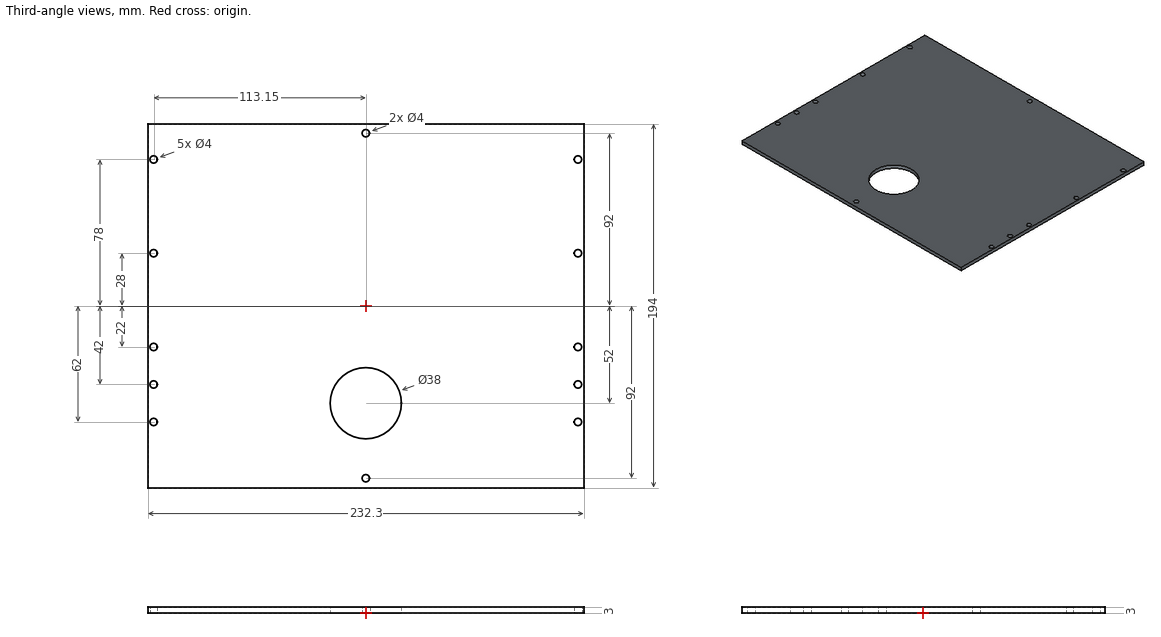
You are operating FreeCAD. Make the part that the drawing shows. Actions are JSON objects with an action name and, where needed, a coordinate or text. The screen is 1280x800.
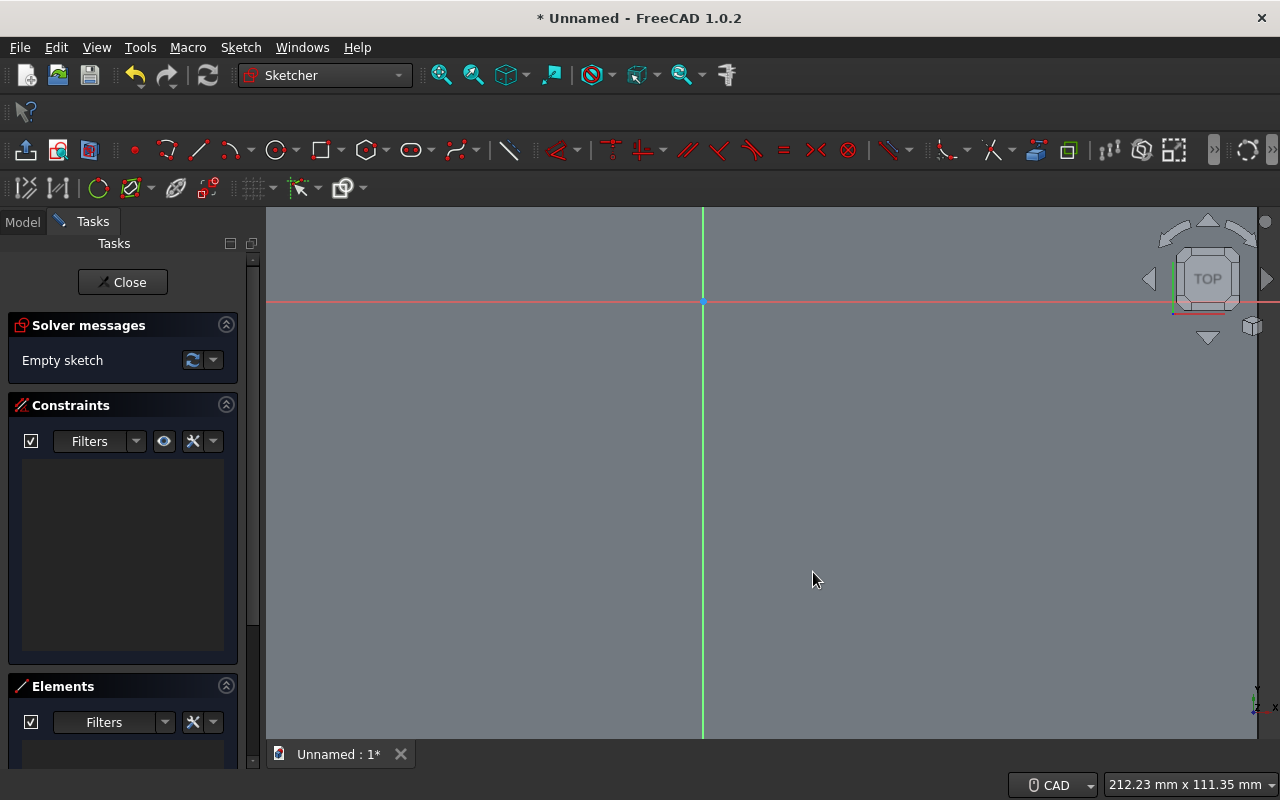
{"action": "left_click", "coordinate": [276, 150]}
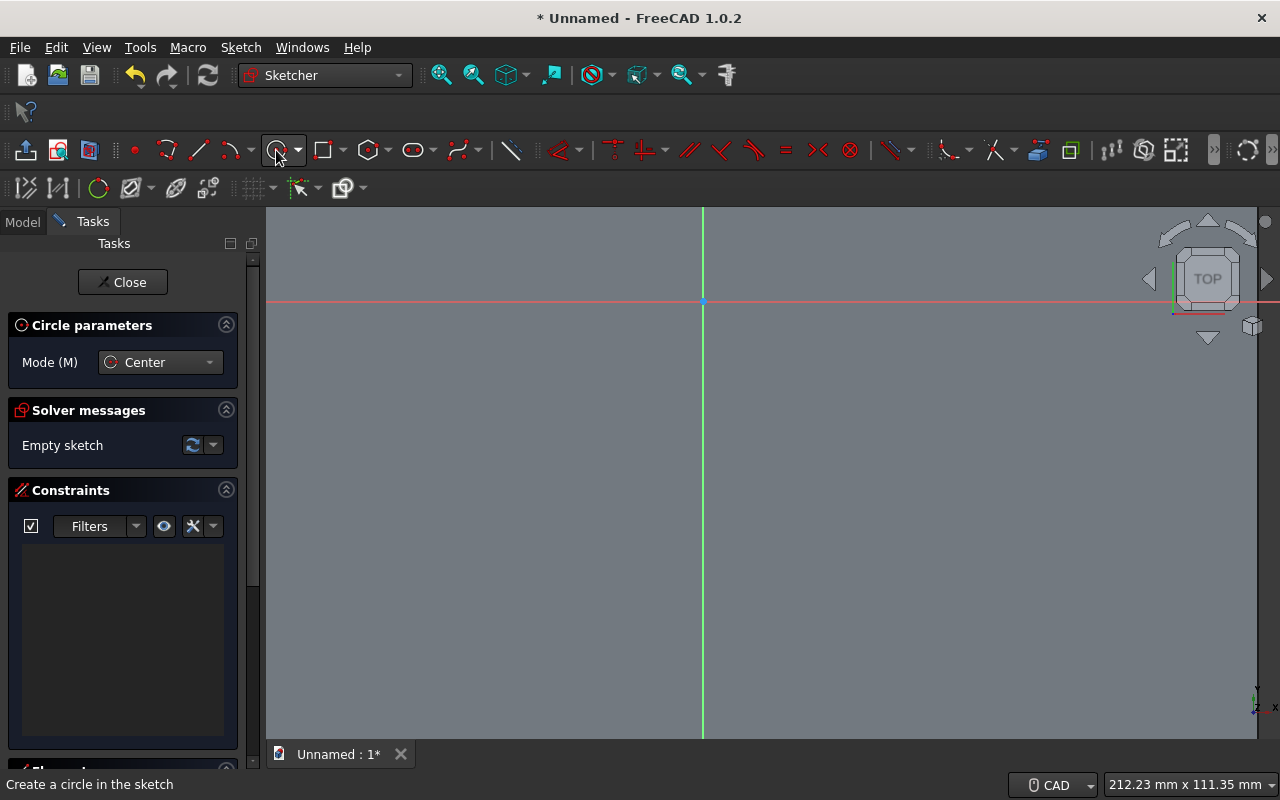
{"action": "left_click", "coordinate": [703, 550]}
{"action": "left_click", "coordinate": [768, 486]}
{"action": "key", "text": "Escape"}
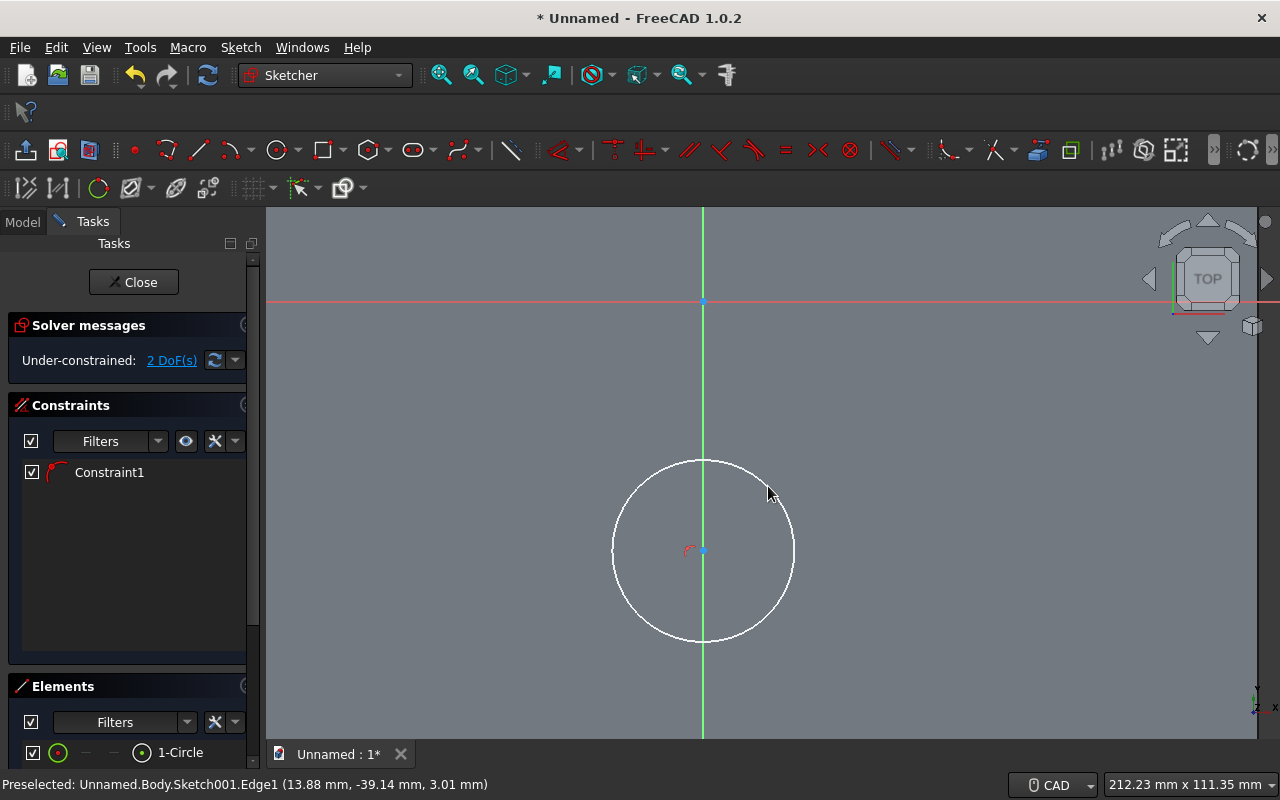
{"action": "key", "text": "d"}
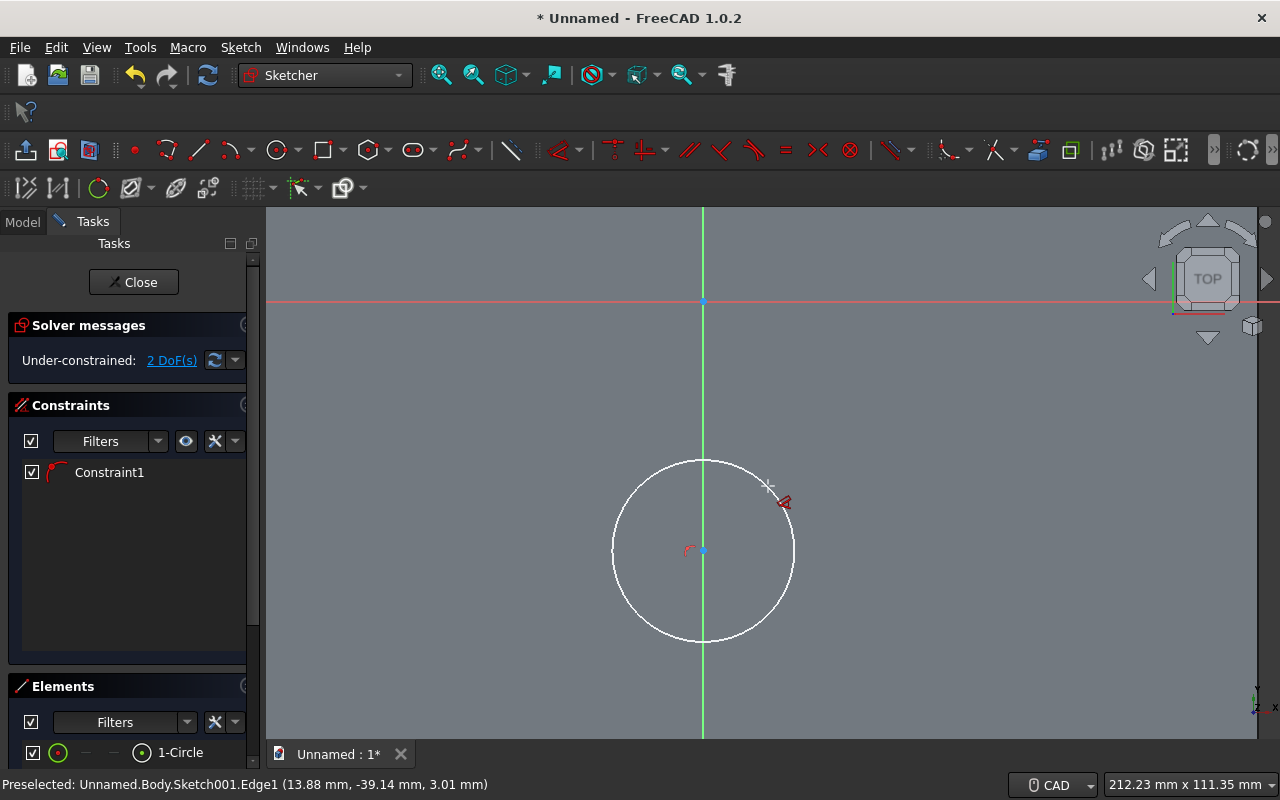
{"action": "left_click", "coordinate": [767, 486]}
{"action": "left_click", "coordinate": [789, 463]}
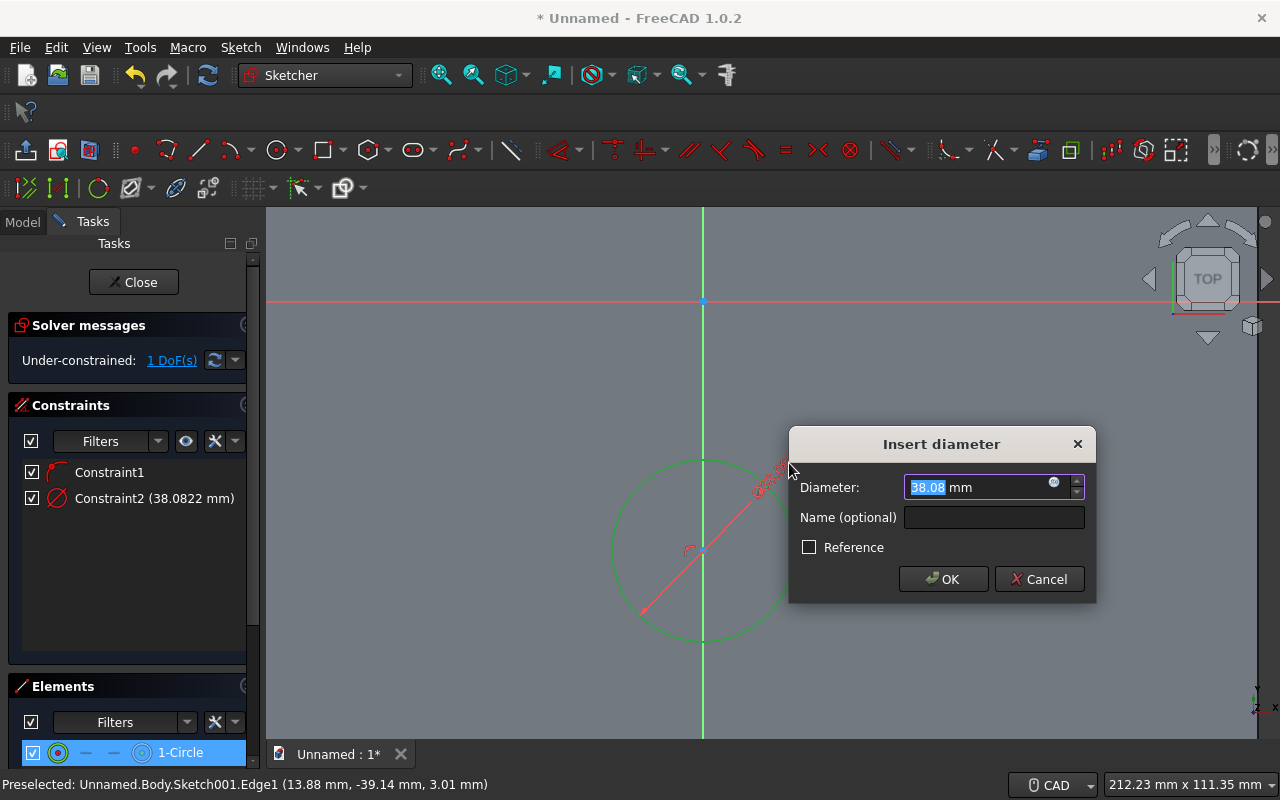
{"action": "type", "text": "38"}
{"action": "key", "text": "Return"}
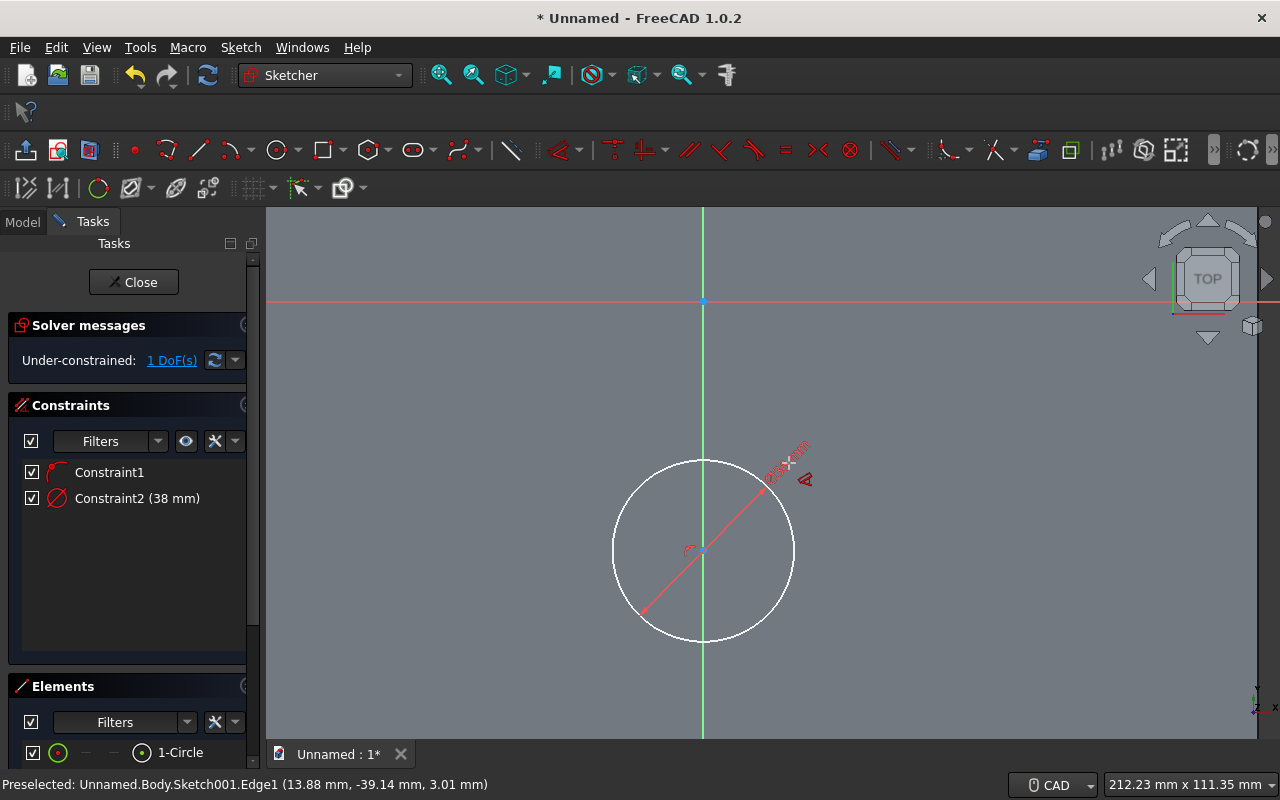
{"action": "left_click", "coordinate": [703, 551]}
{"action": "left_click", "coordinate": [737, 426]}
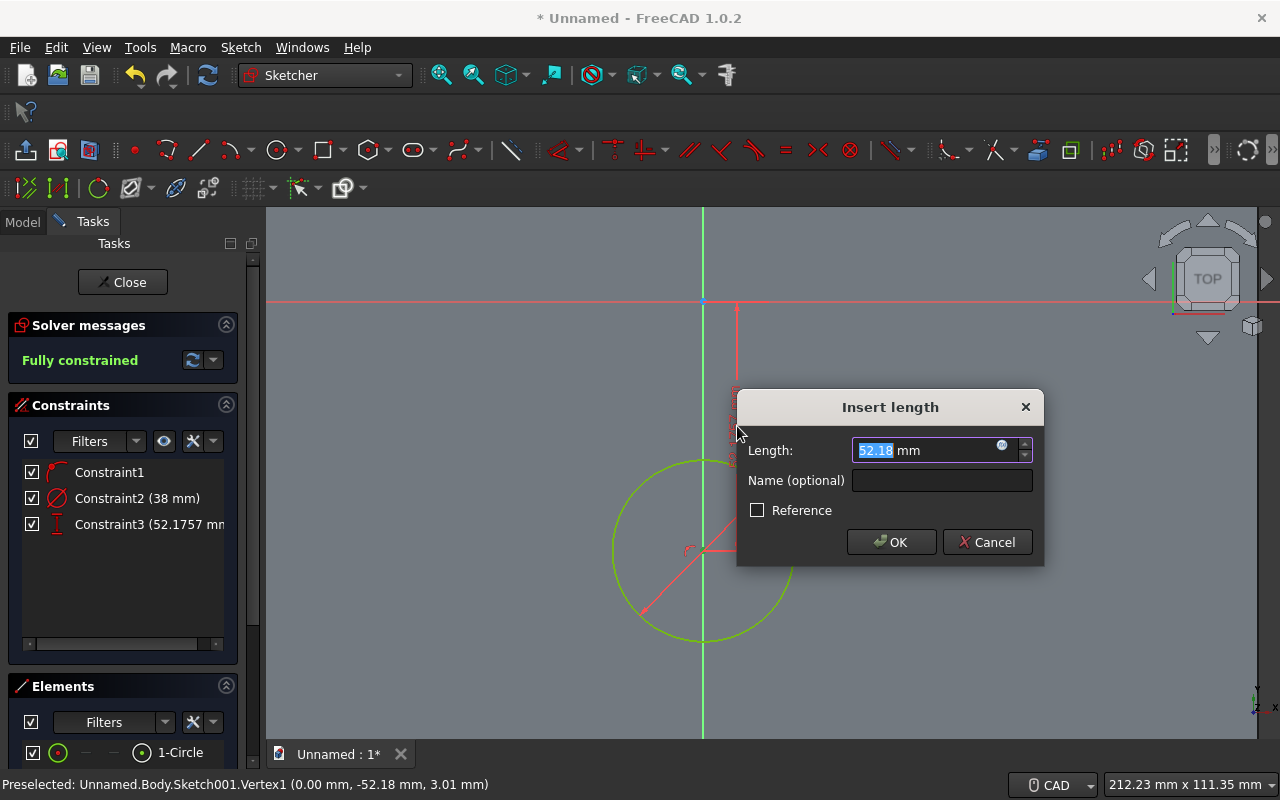
{"action": "type", "text": "52"}
{"action": "key", "text": "Return"}
{"action": "key", "text": "Escape"}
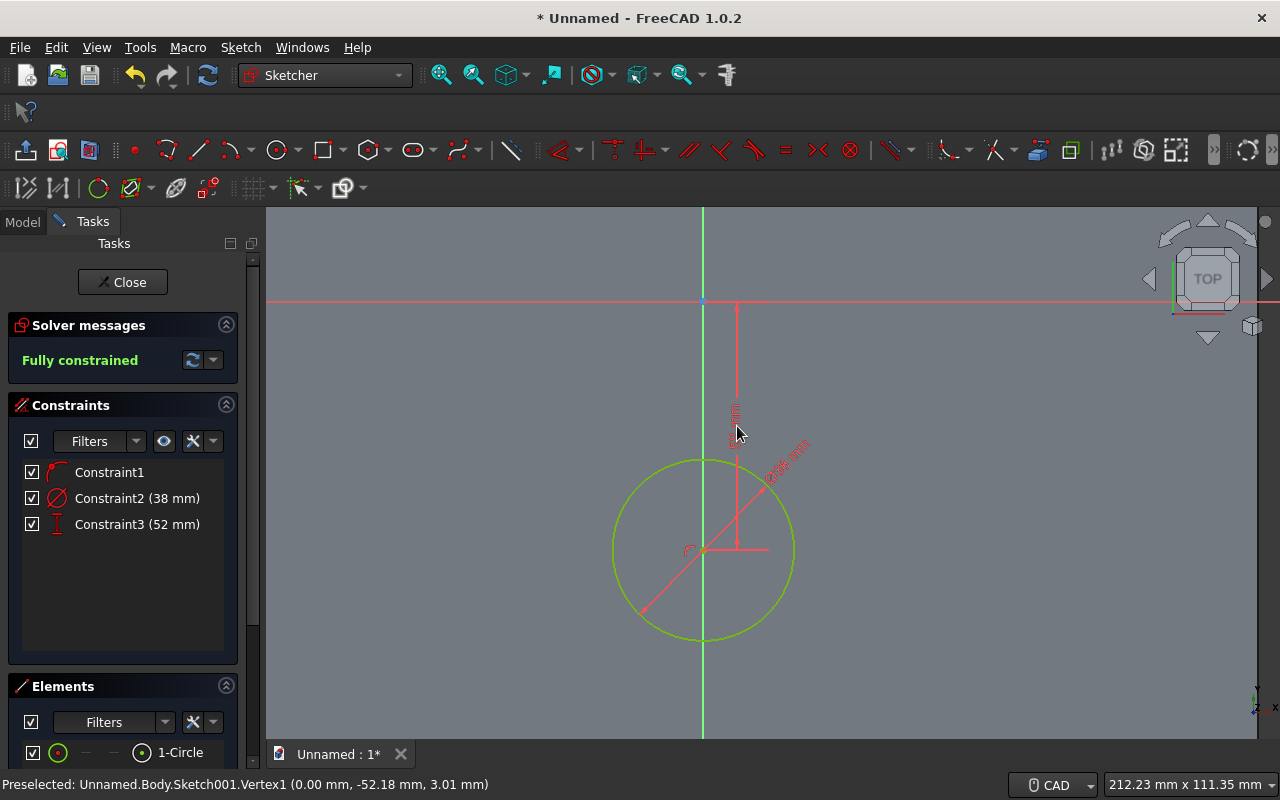
{"action": "left_click", "coordinate": [123, 282]}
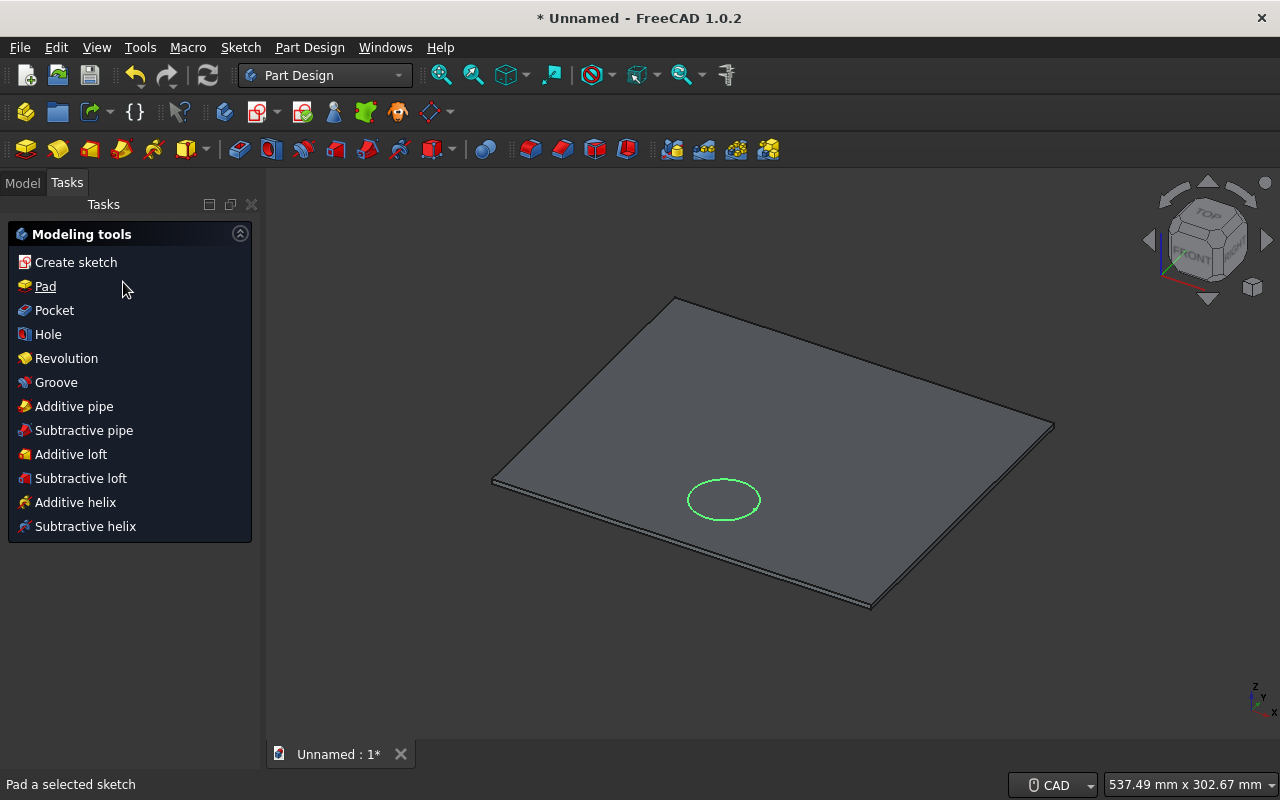
{"action": "left_click", "coordinate": [240, 150]}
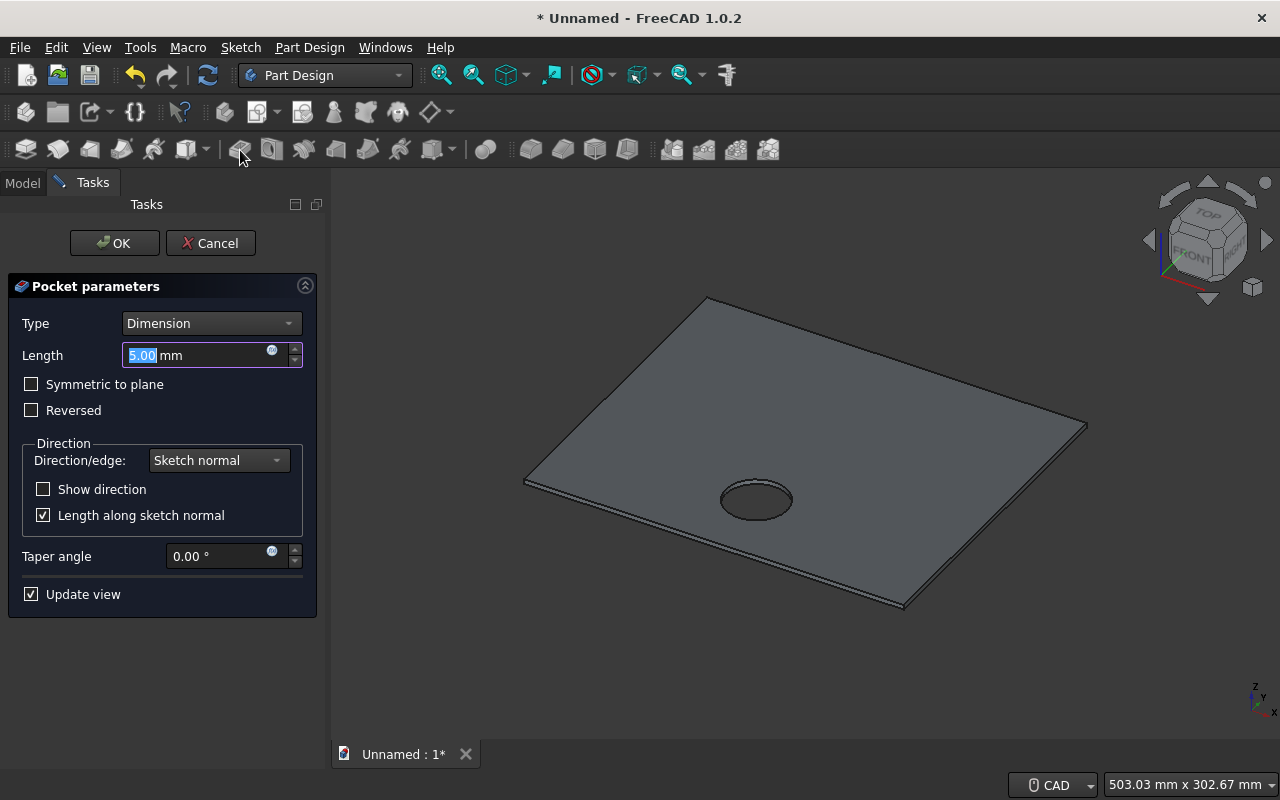
{"action": "type", "text": "3"}
{"action": "key", "text": "Tab"}